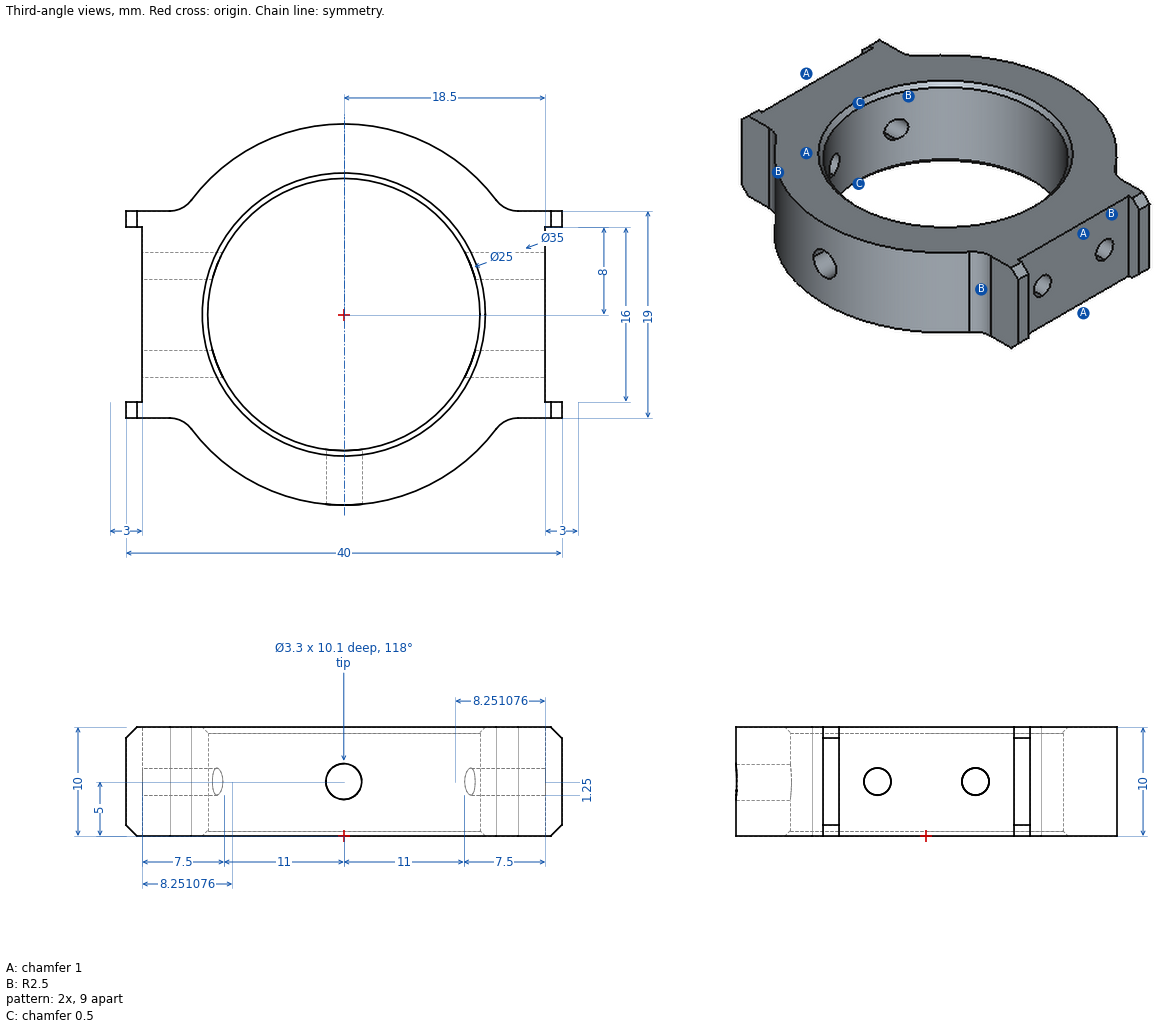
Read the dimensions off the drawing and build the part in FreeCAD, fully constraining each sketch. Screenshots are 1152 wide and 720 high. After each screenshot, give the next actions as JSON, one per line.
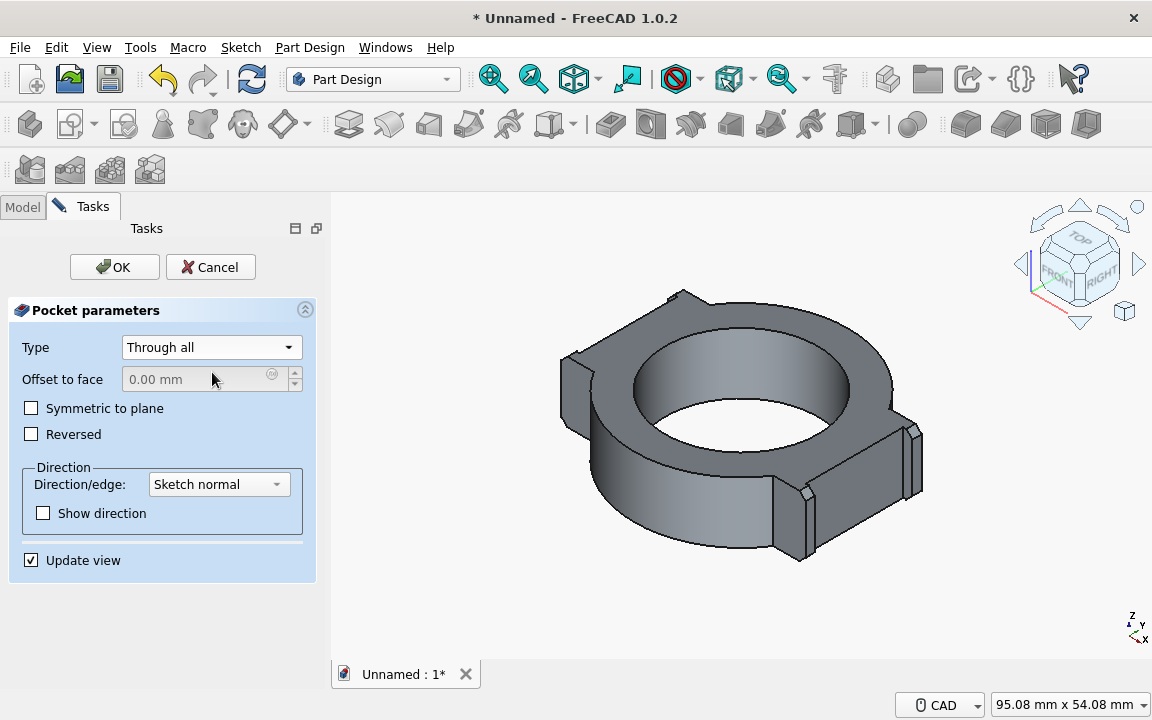
{"action": "left_click", "coordinate": [115, 267]}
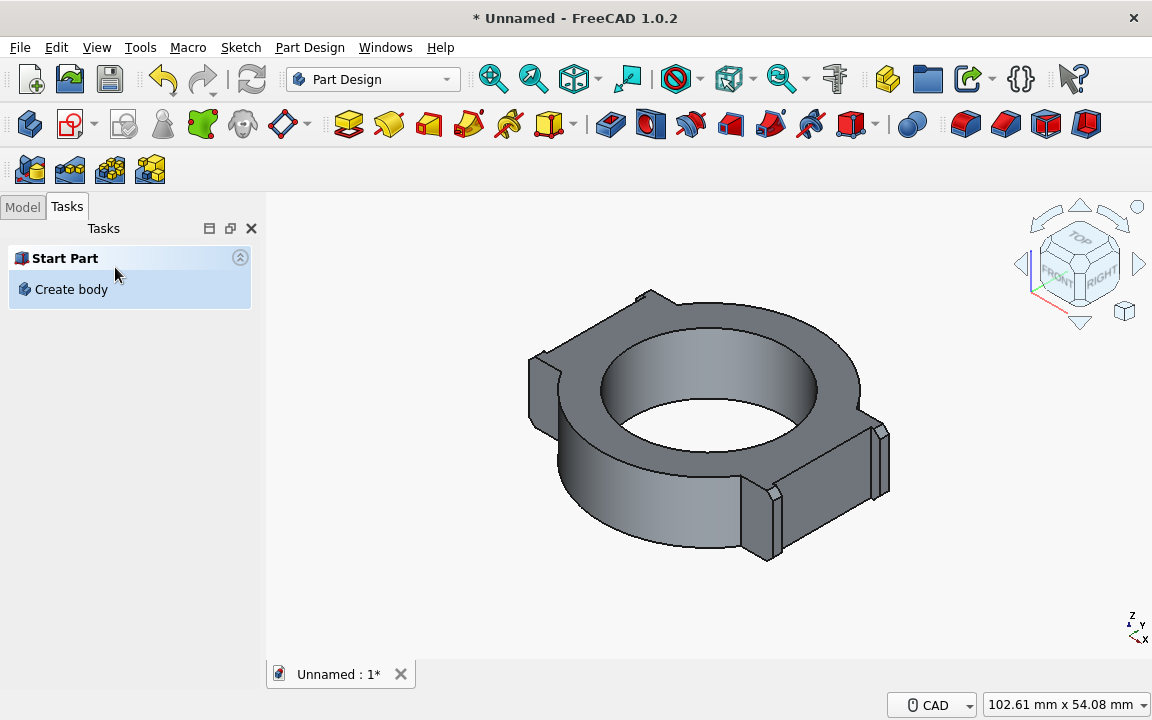
{"action": "left_click", "coordinate": [23, 206]}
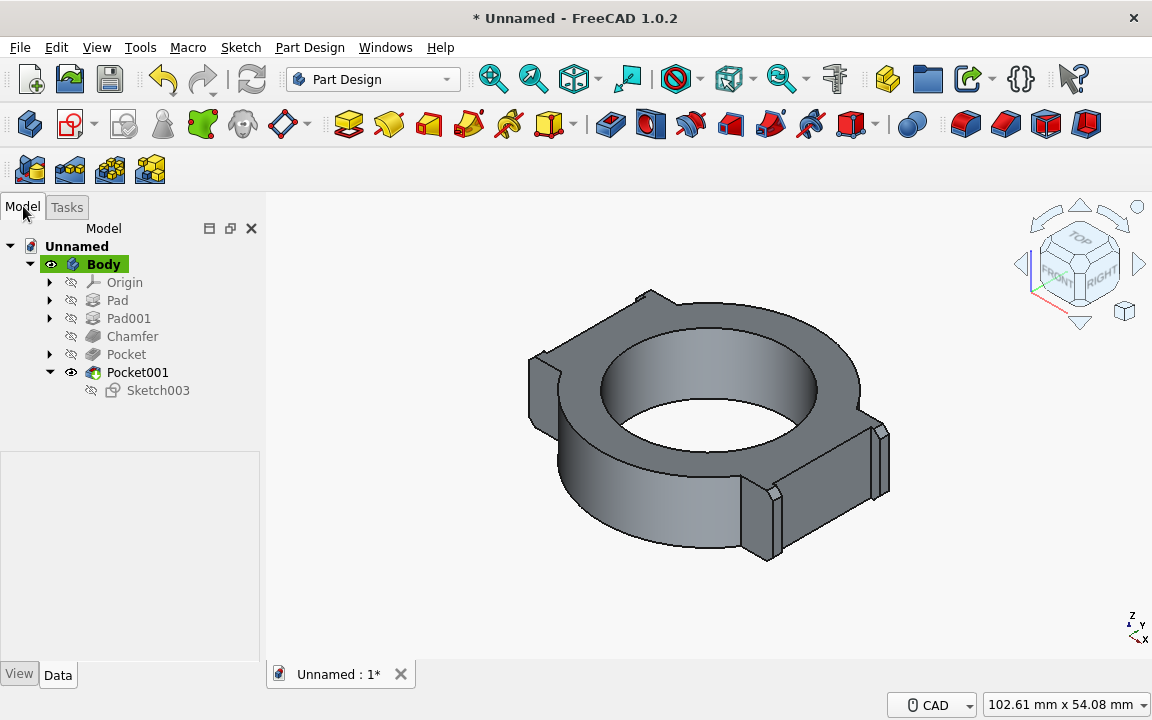
{"action": "left_click", "coordinate": [50, 282]}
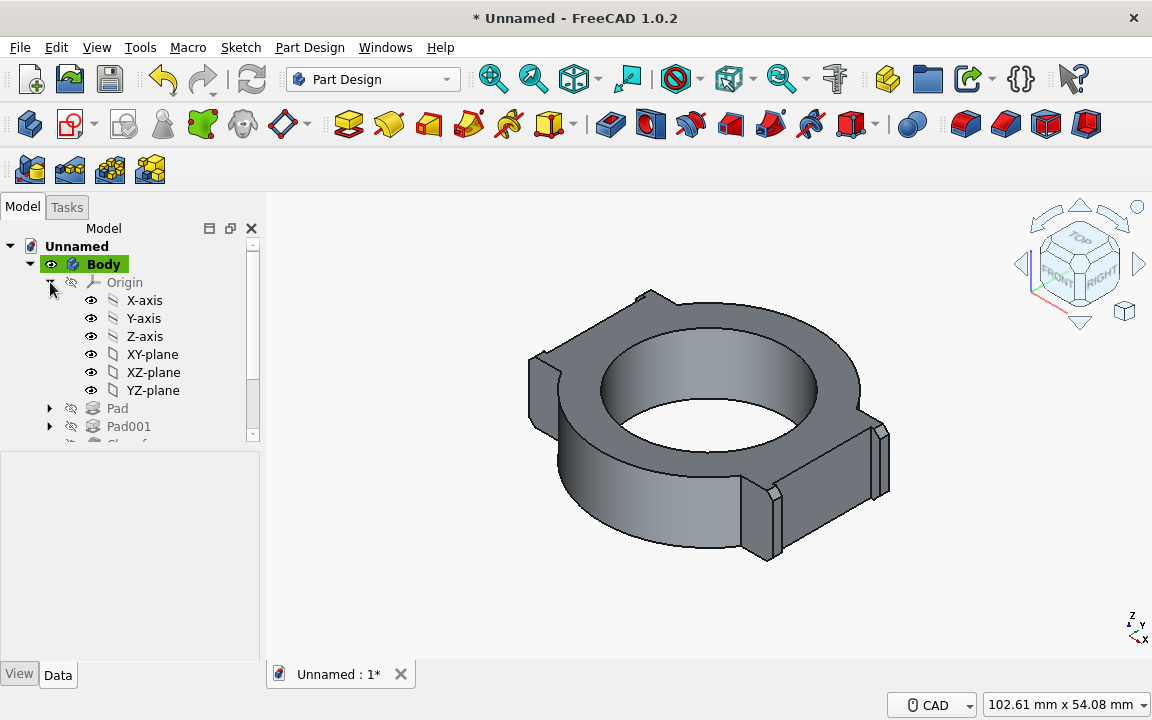
{"action": "left_click", "coordinate": [136, 372]}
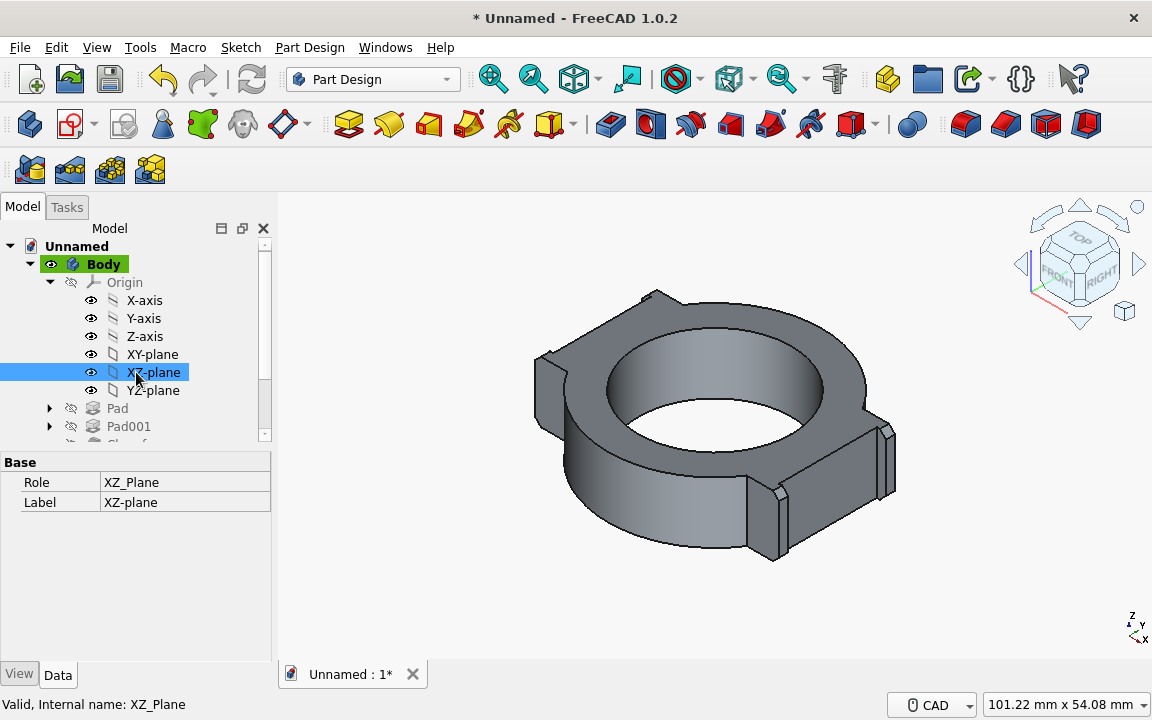
{"action": "left_click", "coordinate": [284, 124]}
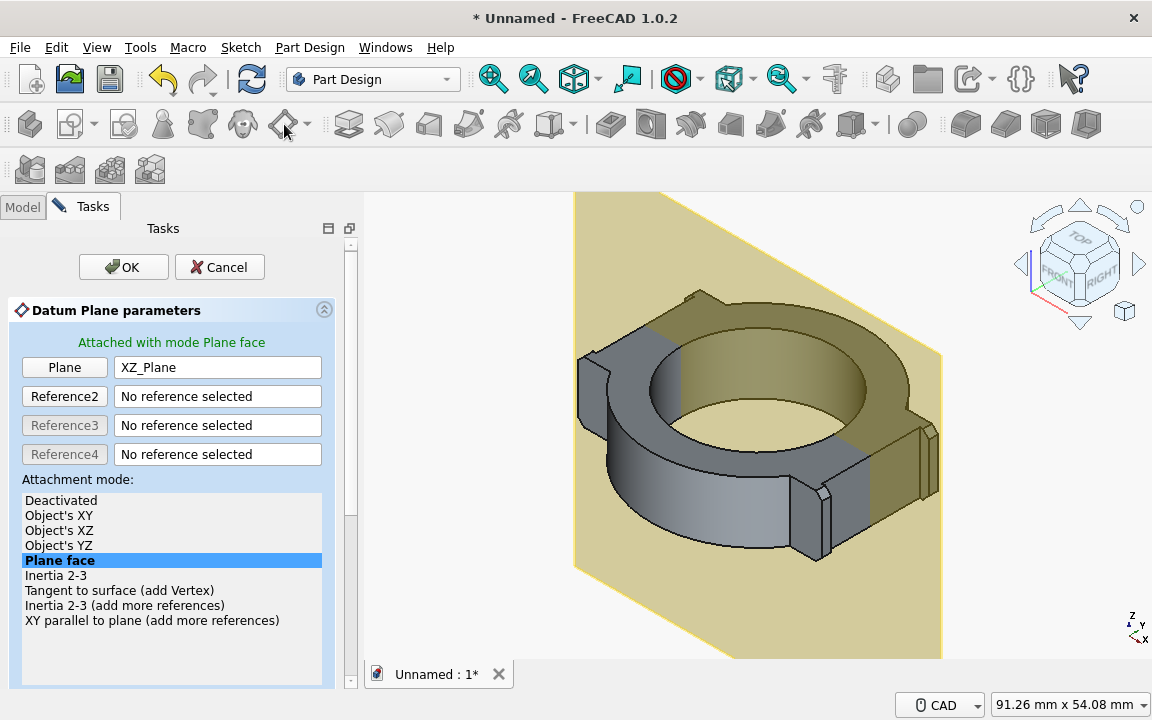
{"action": "scroll", "coordinate": [351, 463], "scroll_direction": "down", "scroll_amount": 3}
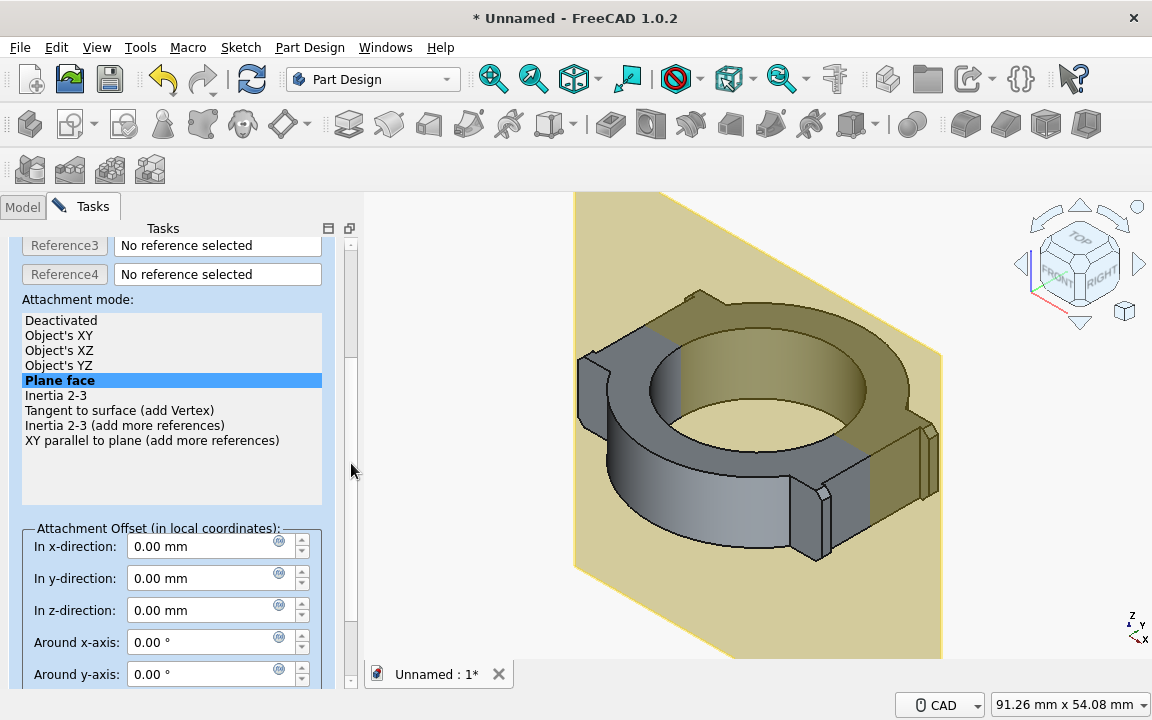
{"action": "triple_click", "coordinate": [210, 610]}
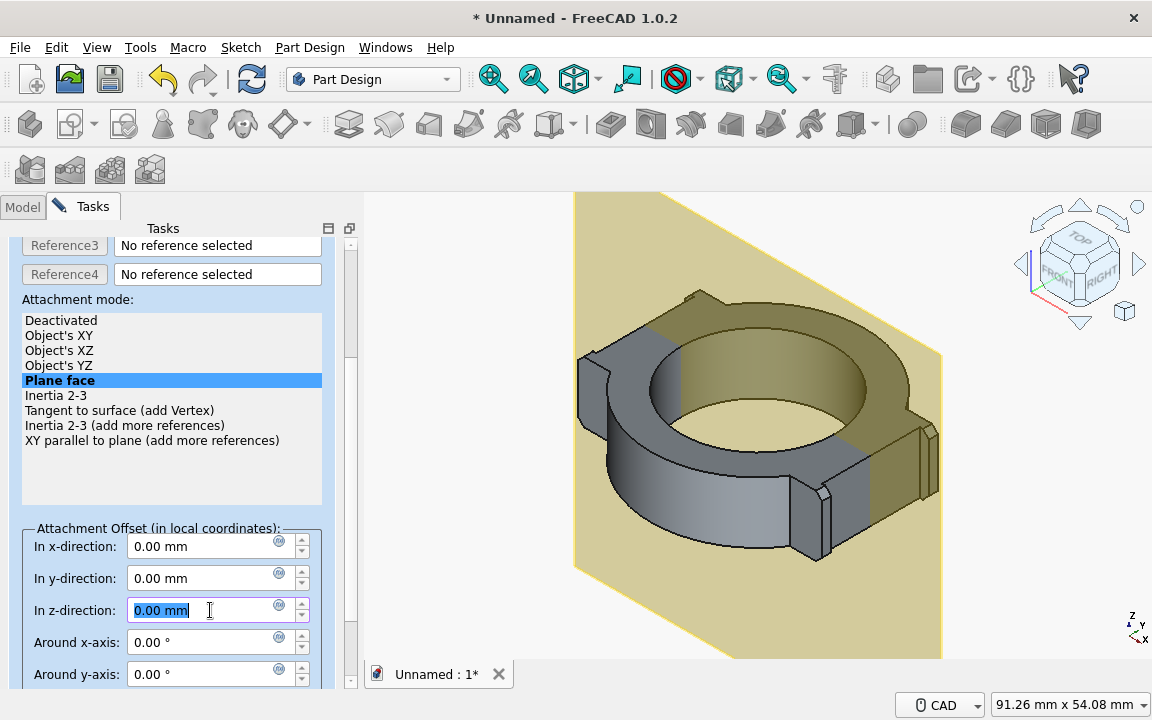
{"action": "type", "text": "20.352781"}
{"action": "key", "text": "Tab"}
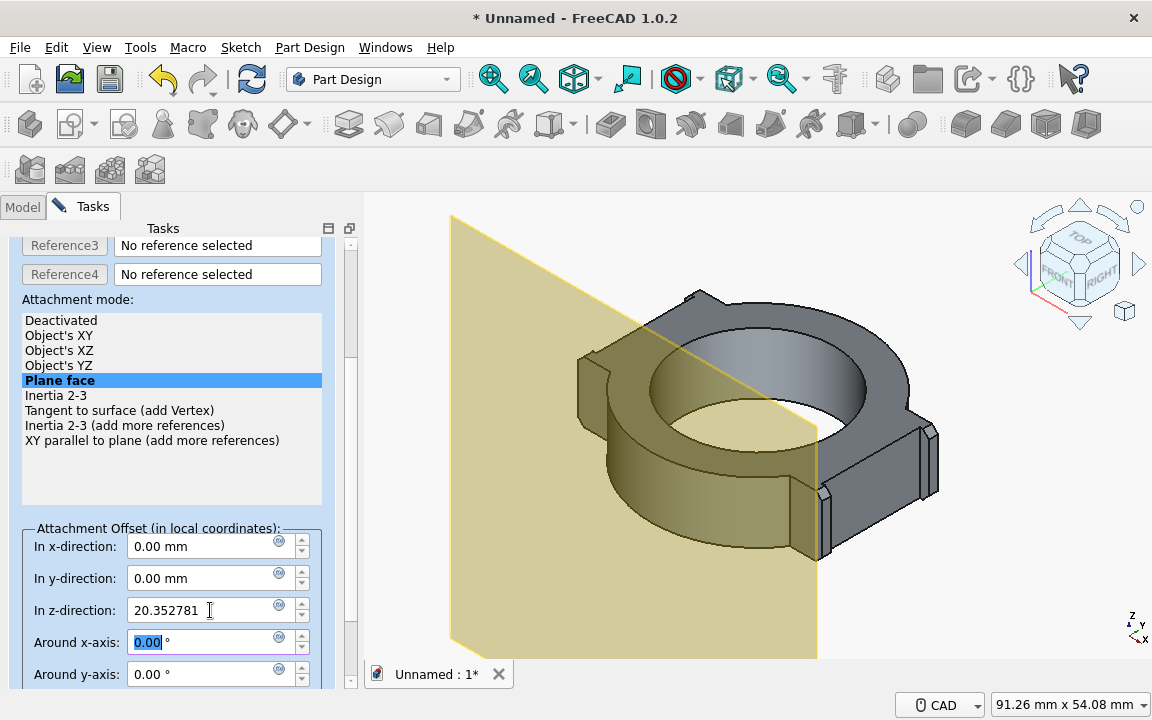
{"action": "scroll", "coordinate": [351, 463], "scroll_direction": "up", "scroll_amount": 4}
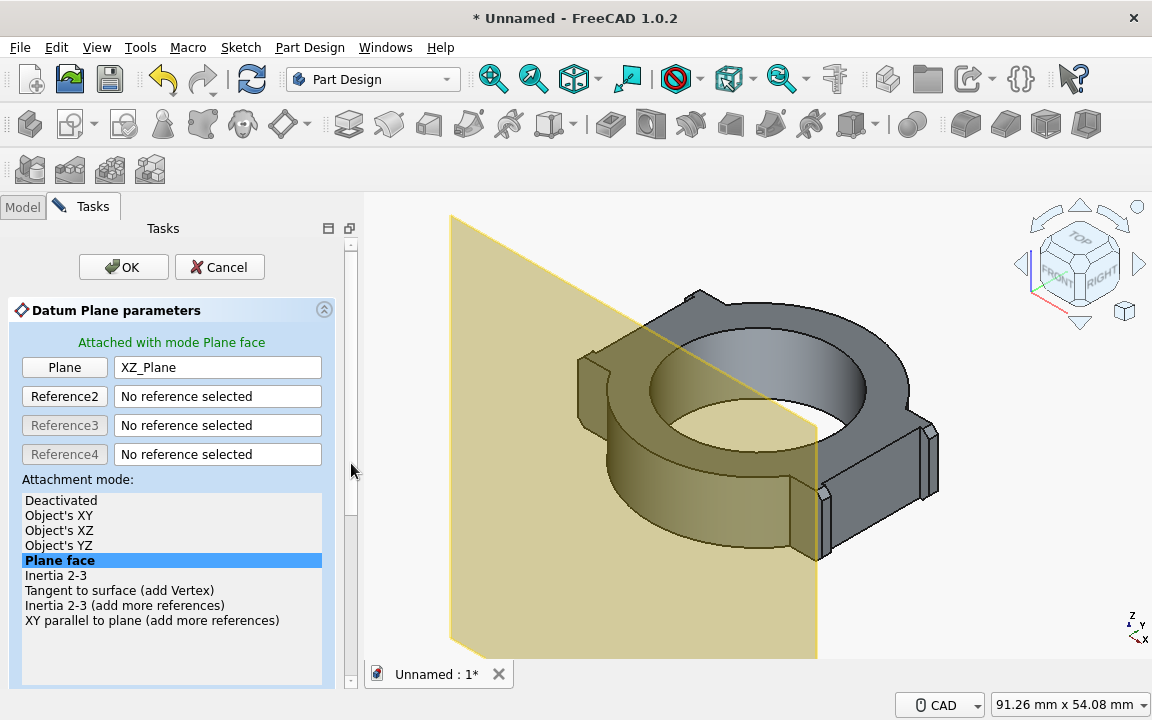
{"action": "left_click", "coordinate": [124, 267]}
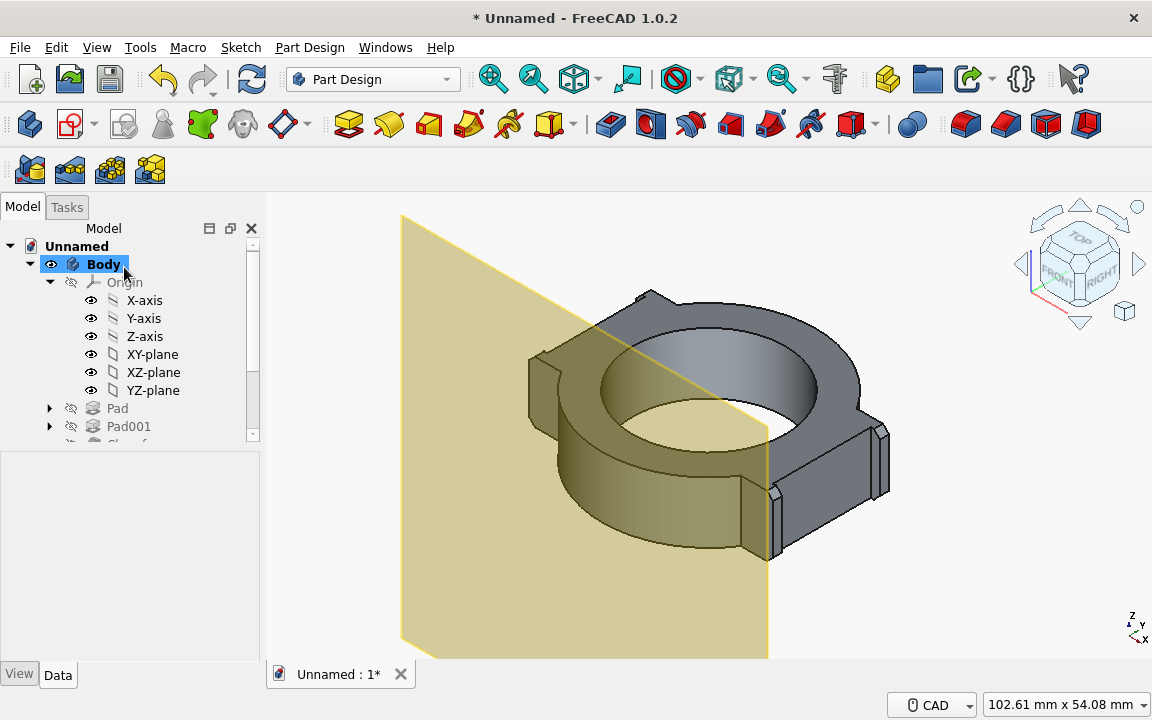
{"action": "scroll", "coordinate": [100, 332], "scroll_direction": "down", "scroll_amount": 3}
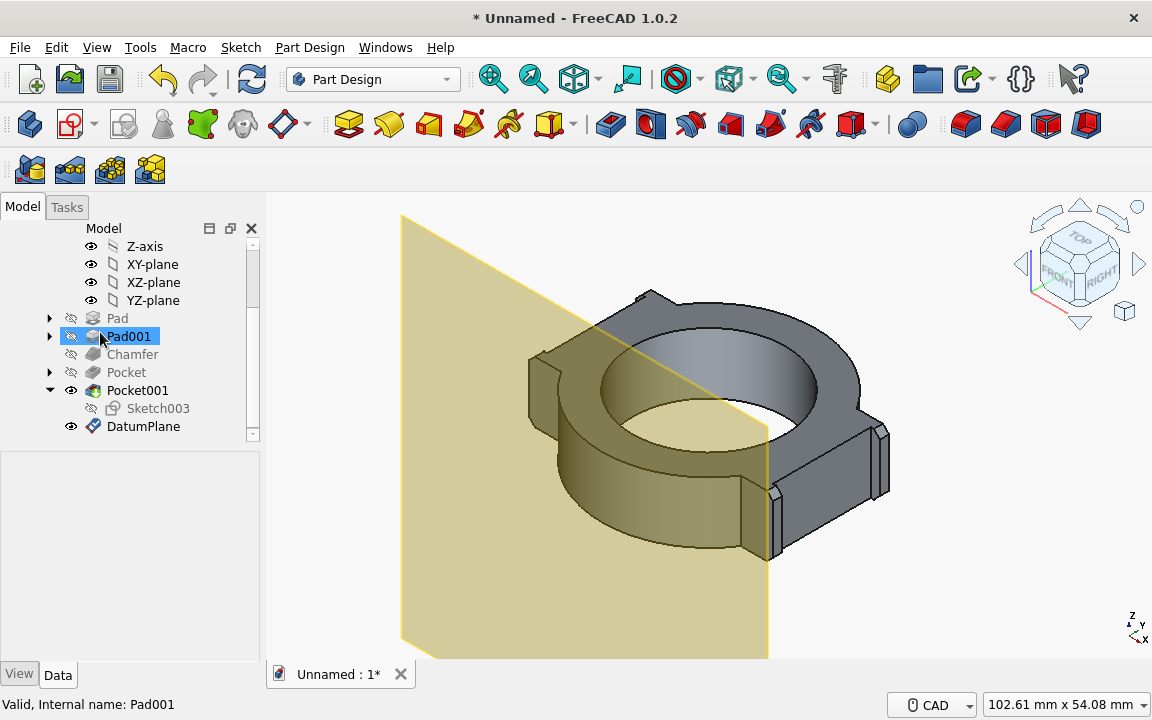
{"action": "left_click", "coordinate": [116, 426]}